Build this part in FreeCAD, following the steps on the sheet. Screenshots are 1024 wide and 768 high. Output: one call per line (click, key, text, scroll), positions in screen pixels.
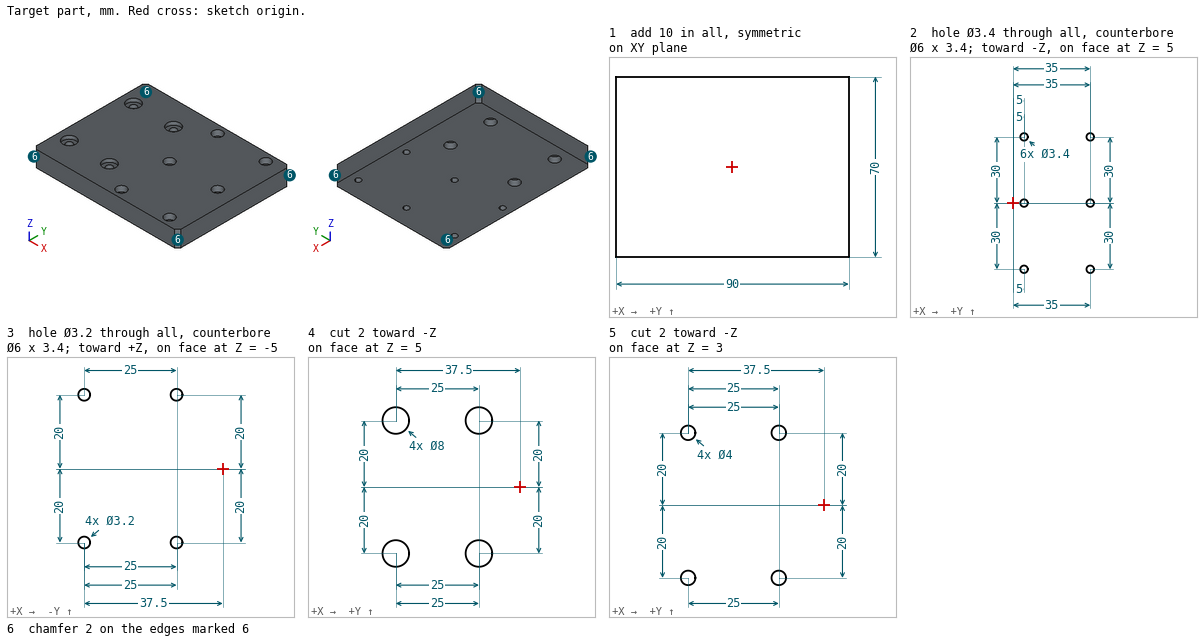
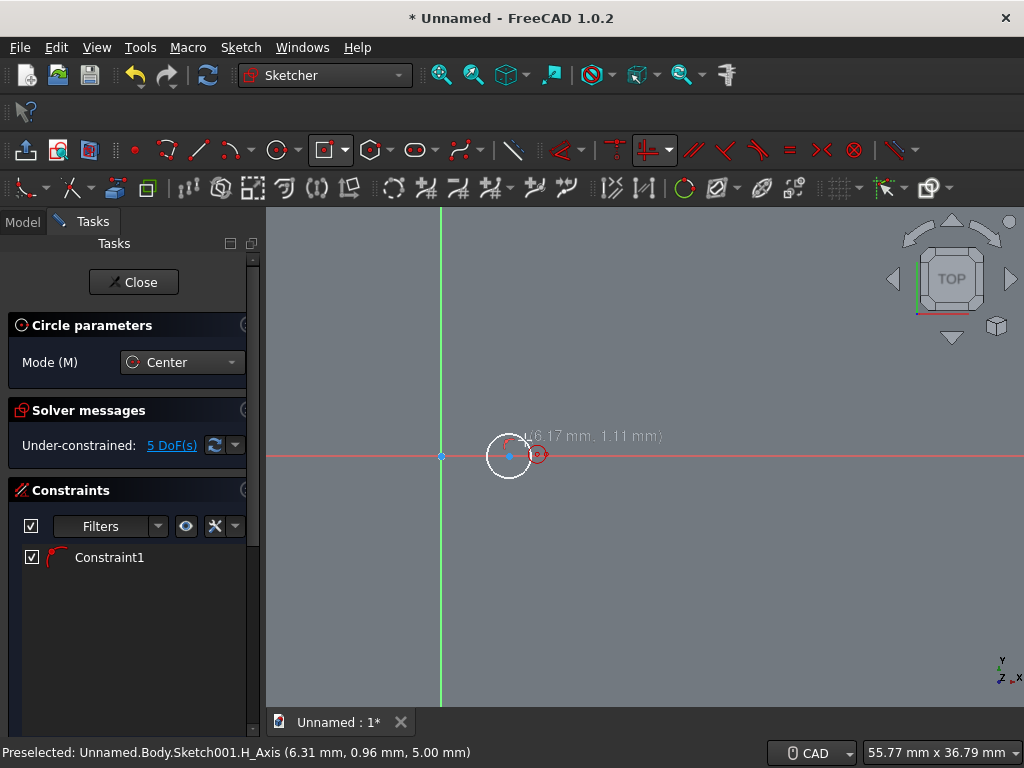
scroll(510, 458, down, 5)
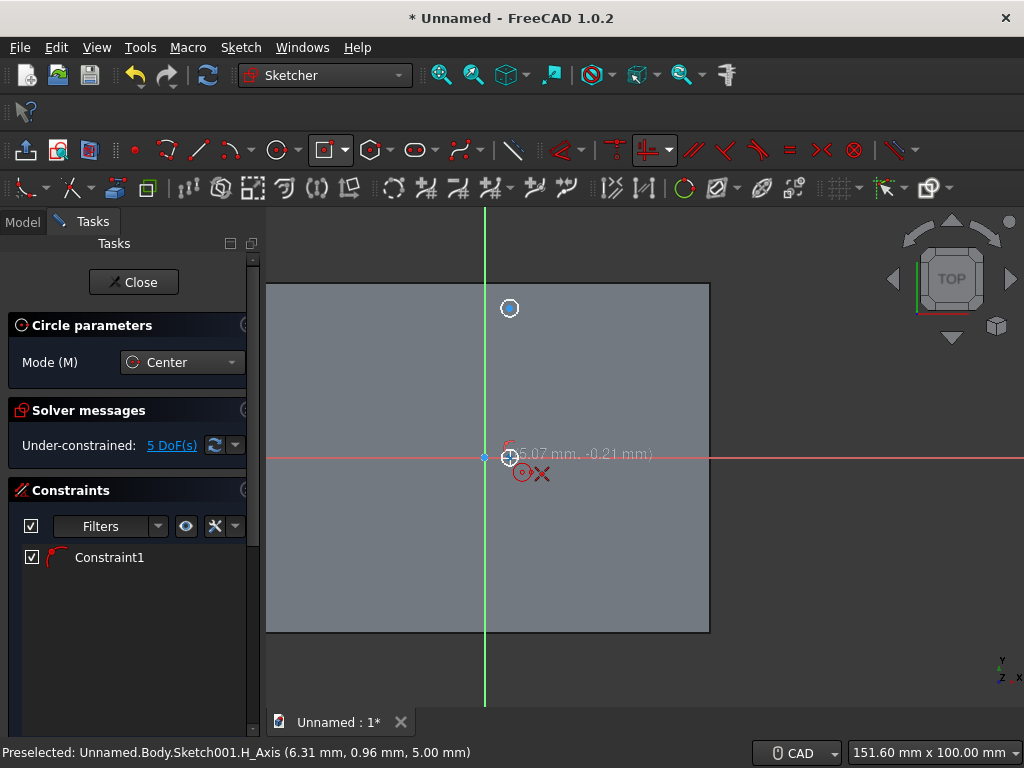
scroll(510, 608, up, 5)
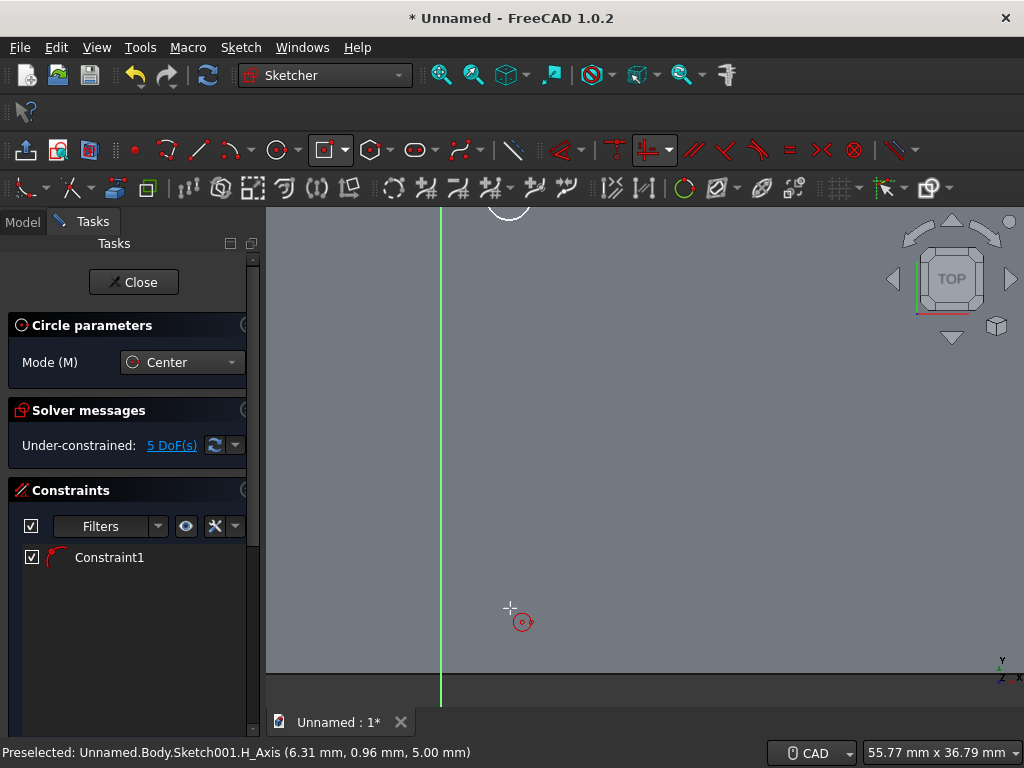
click(509, 606)
click(525, 589)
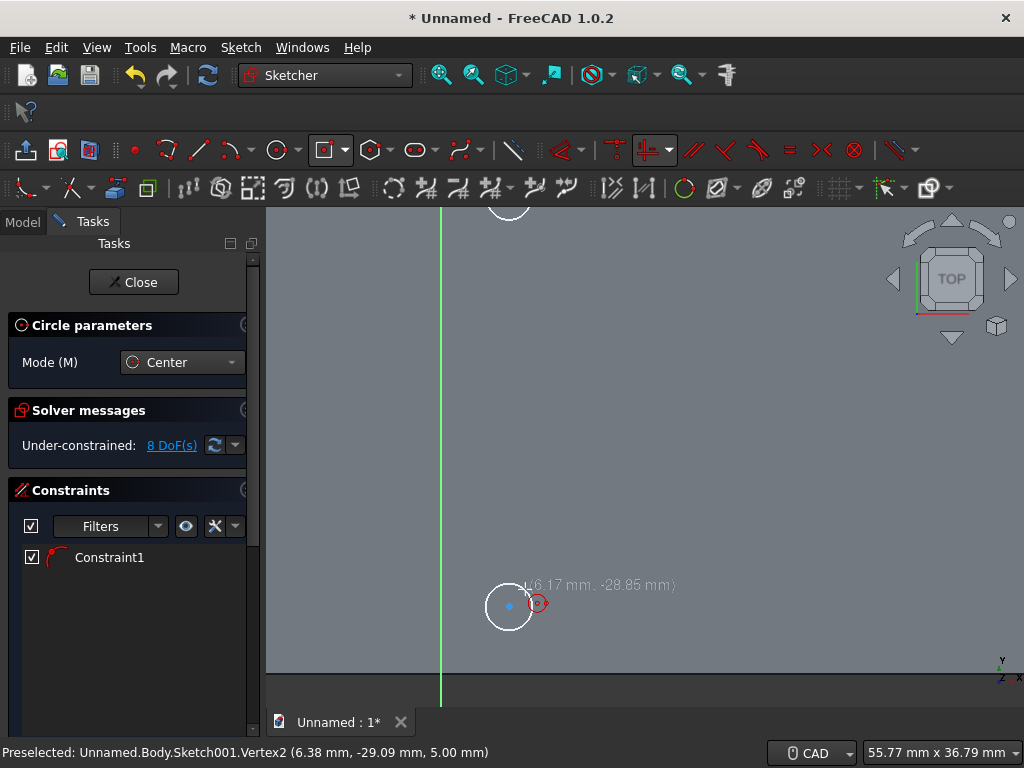
scroll(510, 608, down, 5)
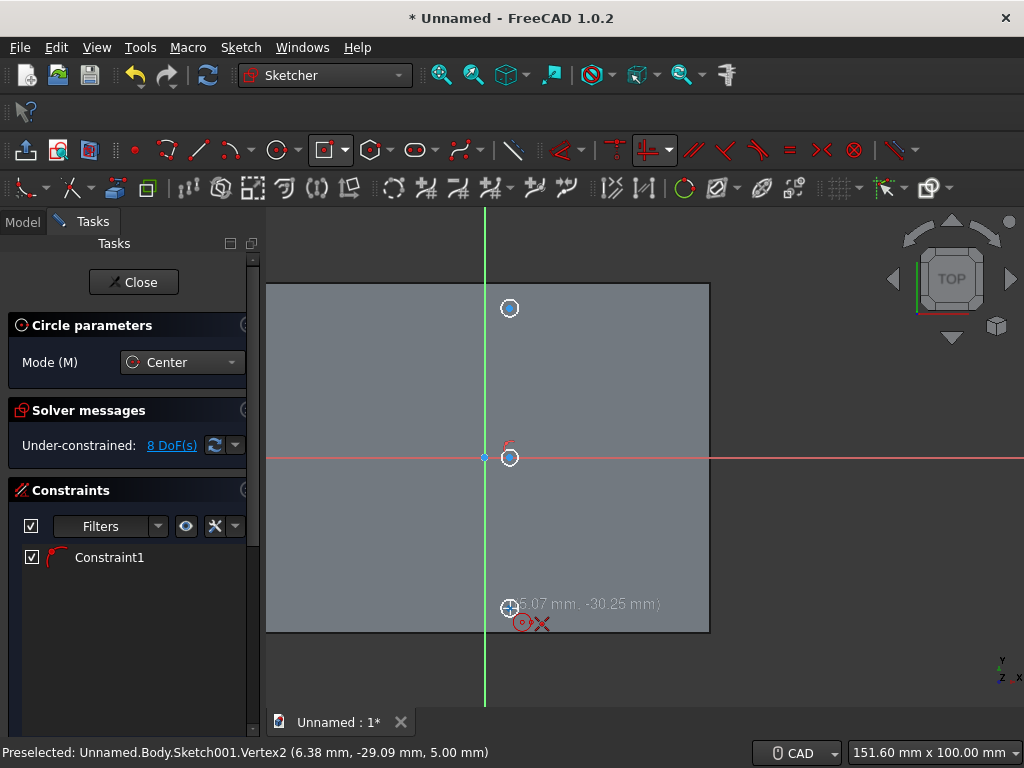
scroll(660, 308, up, 5)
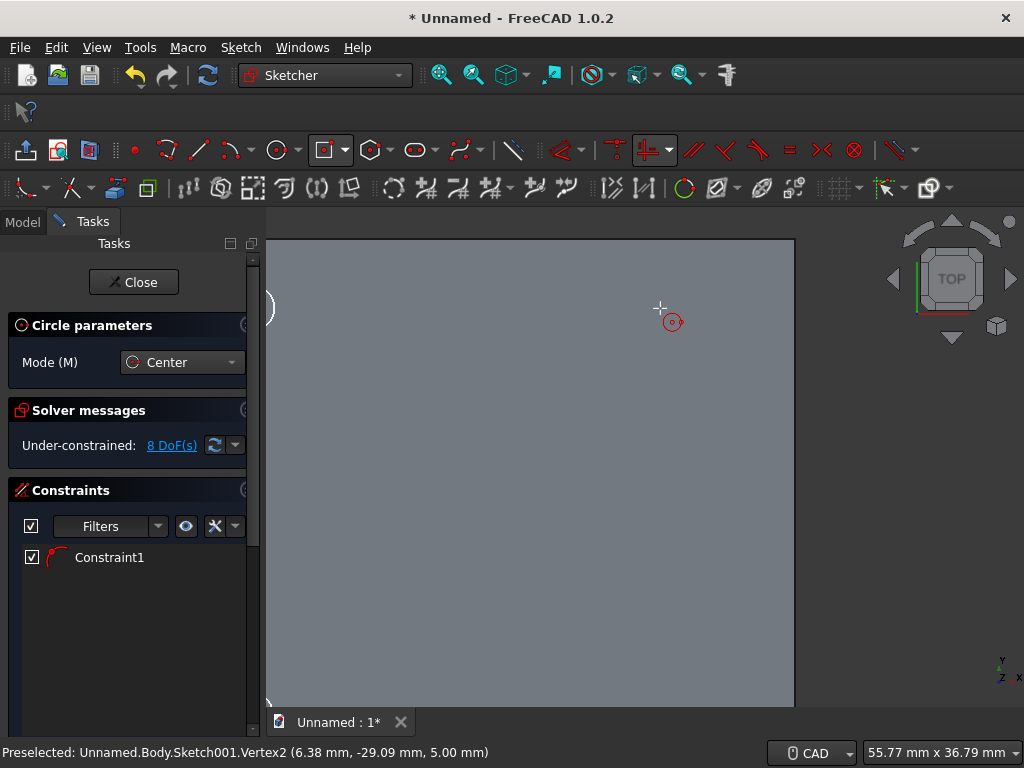
click(659, 307)
click(675, 290)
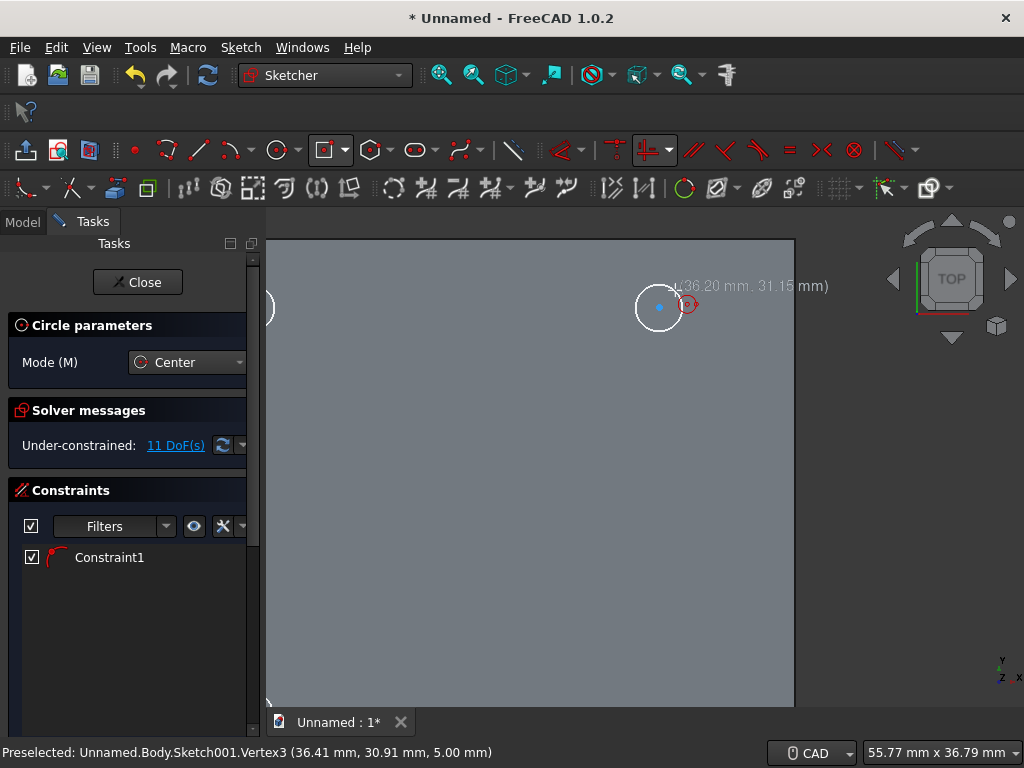
scroll(660, 307, down, 5)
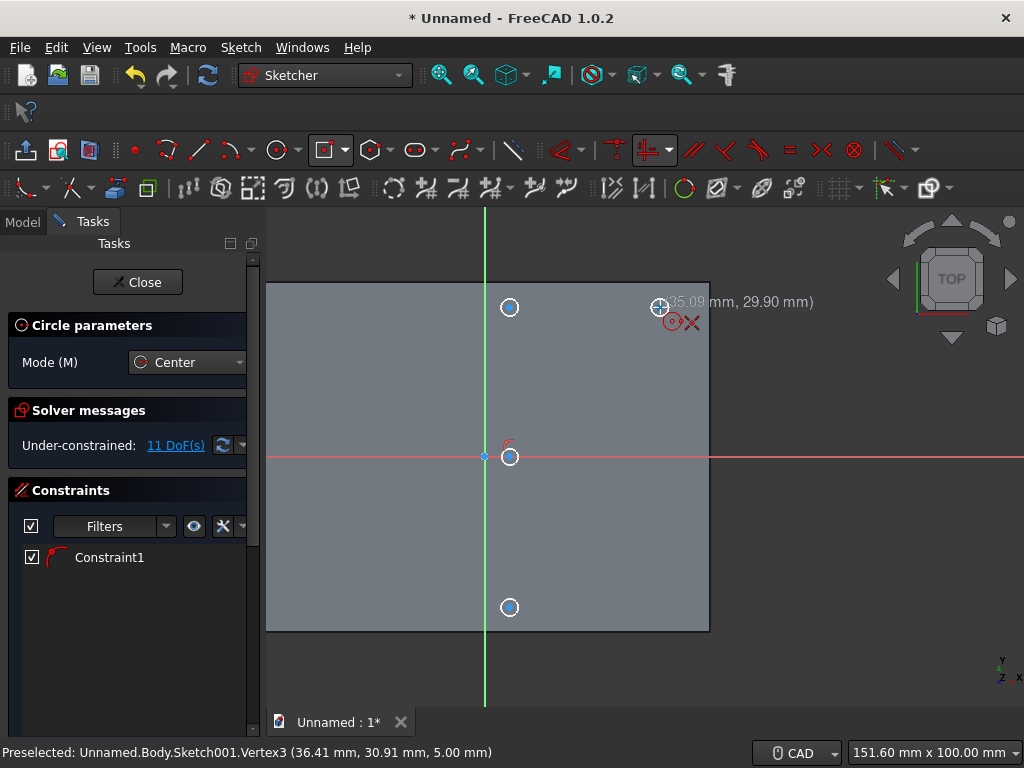
scroll(660, 457, up, 5)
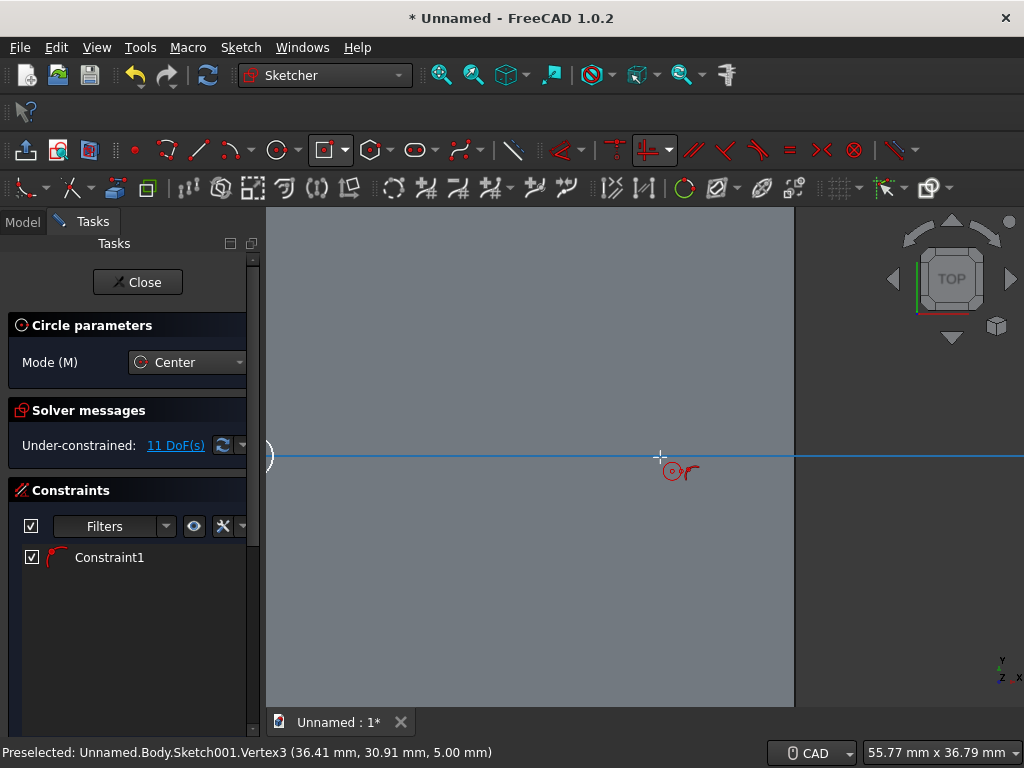
click(659, 456)
click(675, 440)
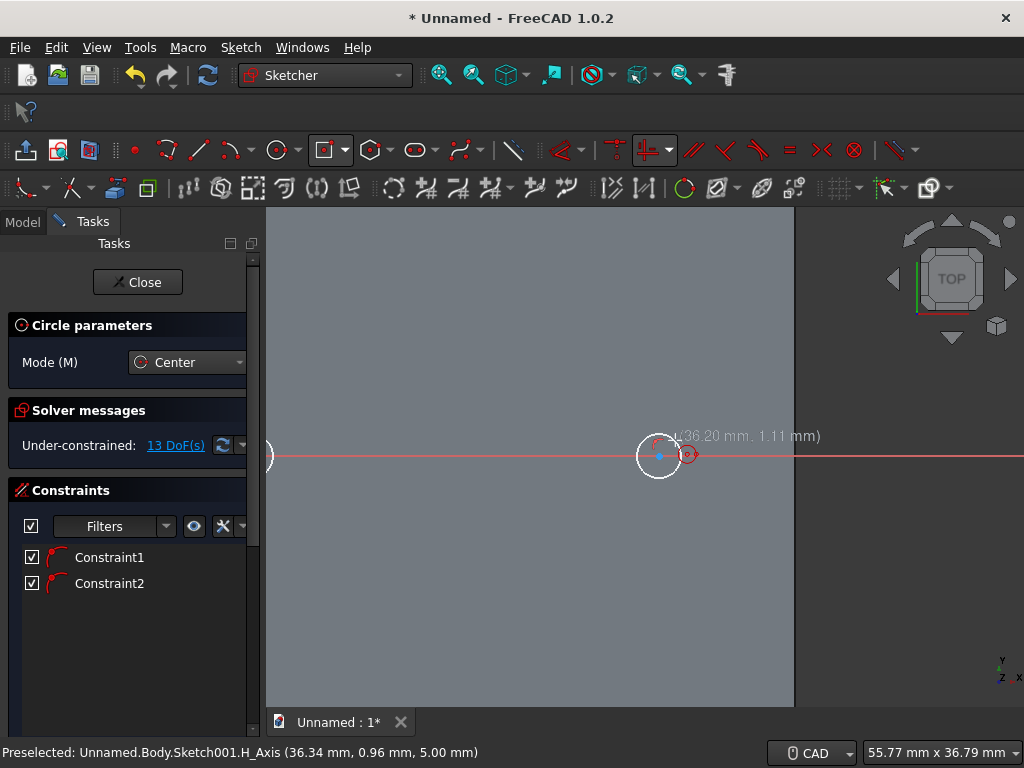
scroll(660, 458, down, 5)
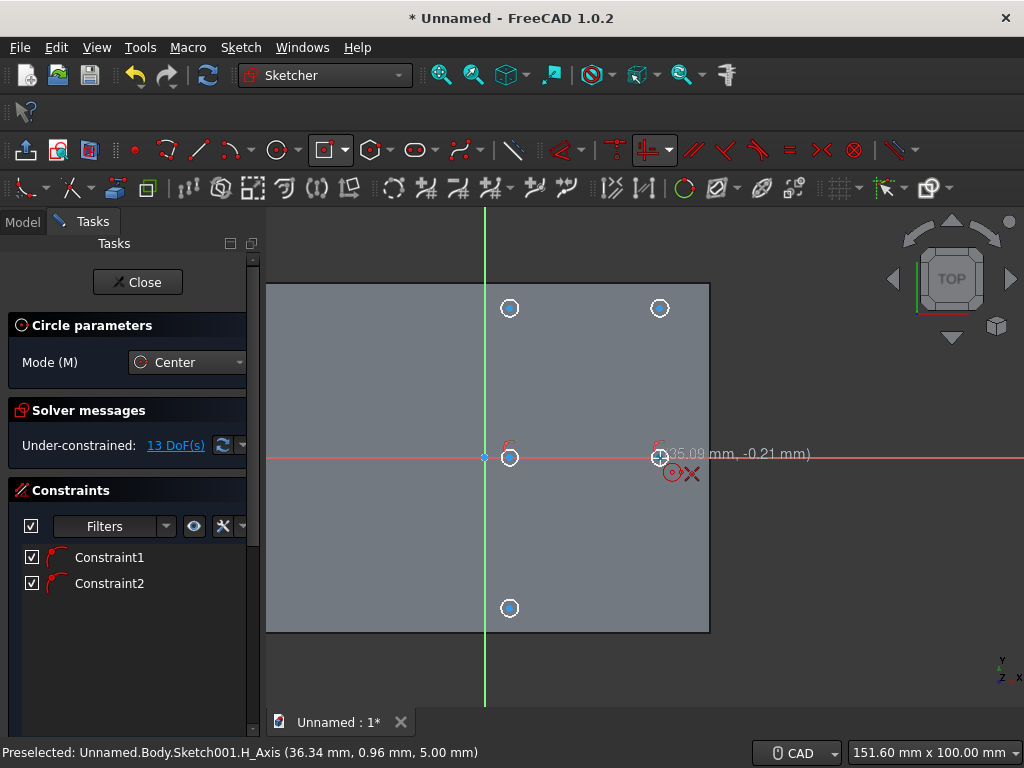
scroll(660, 608, up, 5)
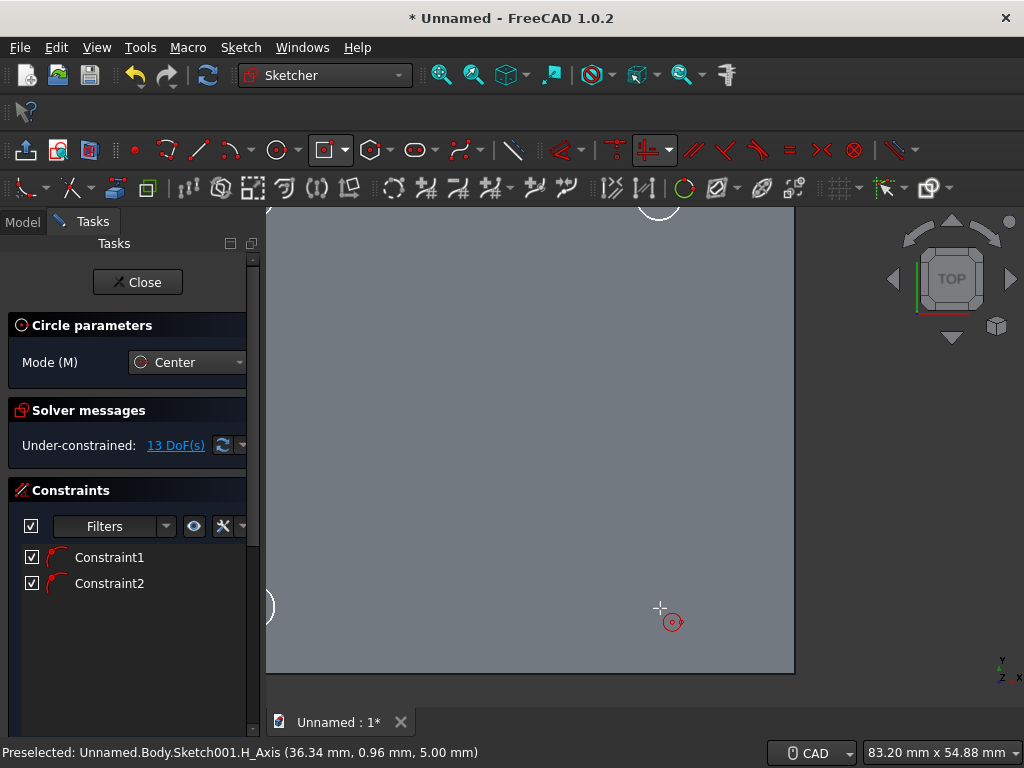
click(659, 606)
click(675, 589)
key(Escape)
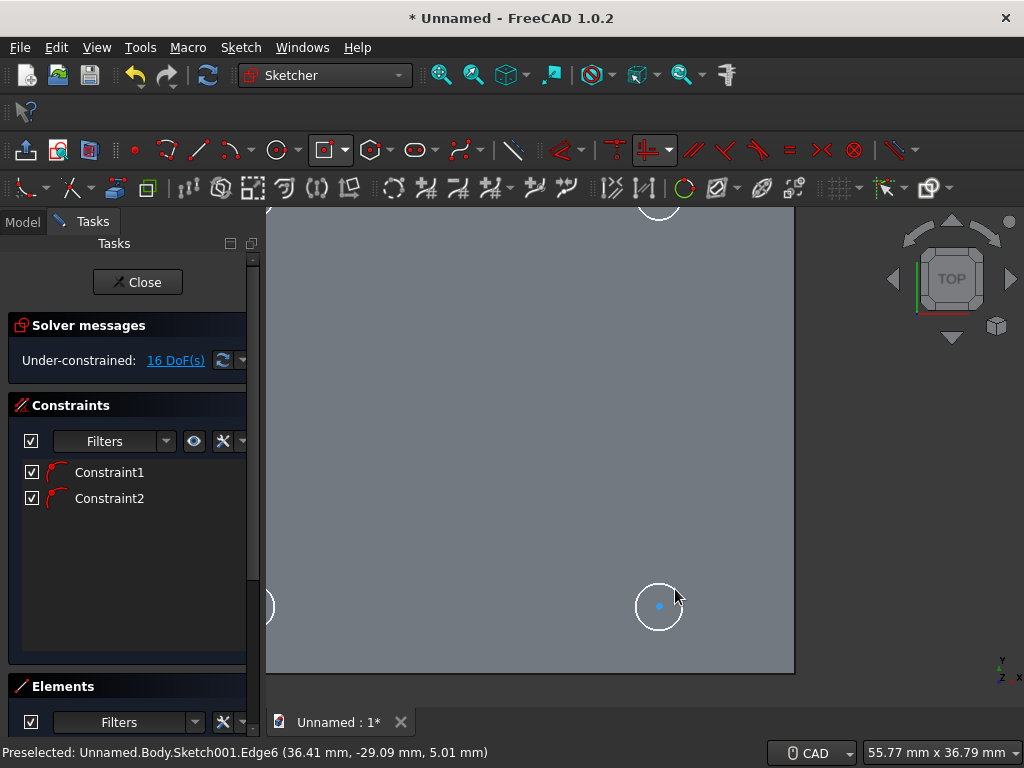
scroll(660, 608, down, 5)